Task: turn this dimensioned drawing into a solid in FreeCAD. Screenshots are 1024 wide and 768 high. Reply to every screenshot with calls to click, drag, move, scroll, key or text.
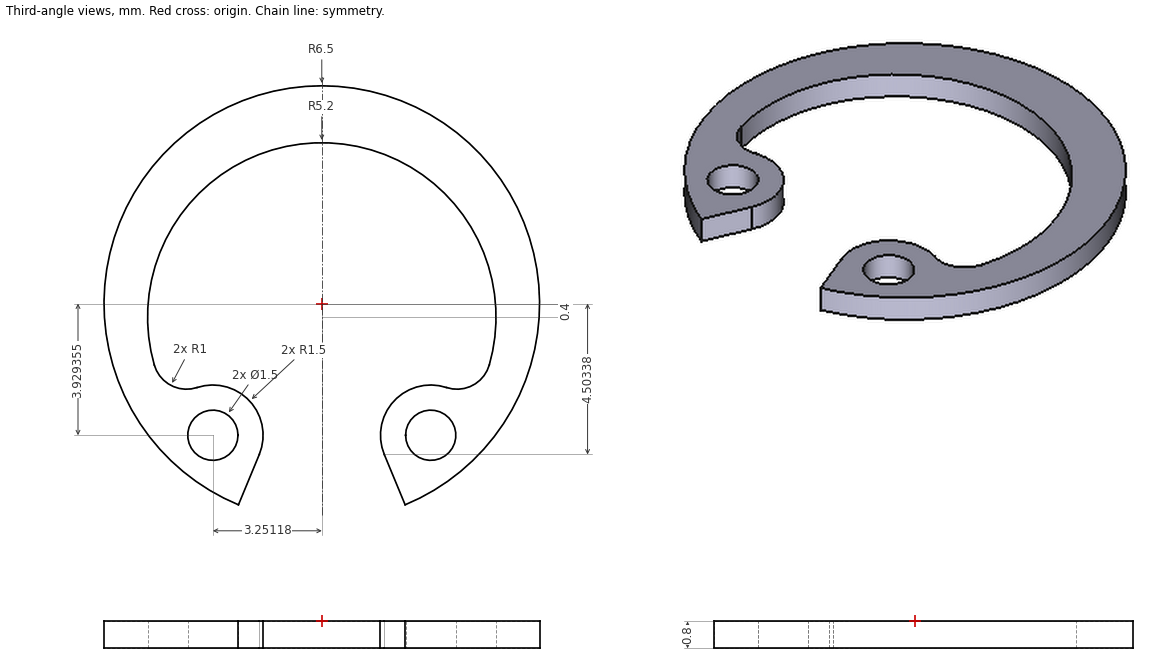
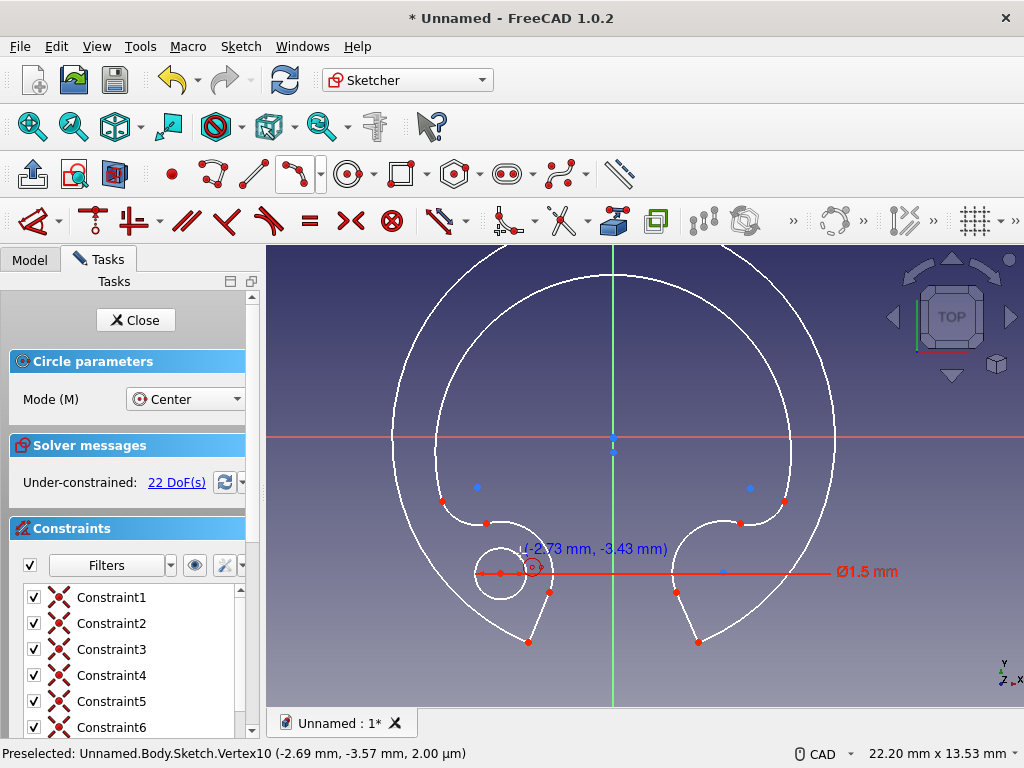
click(724, 571)
move(742, 553)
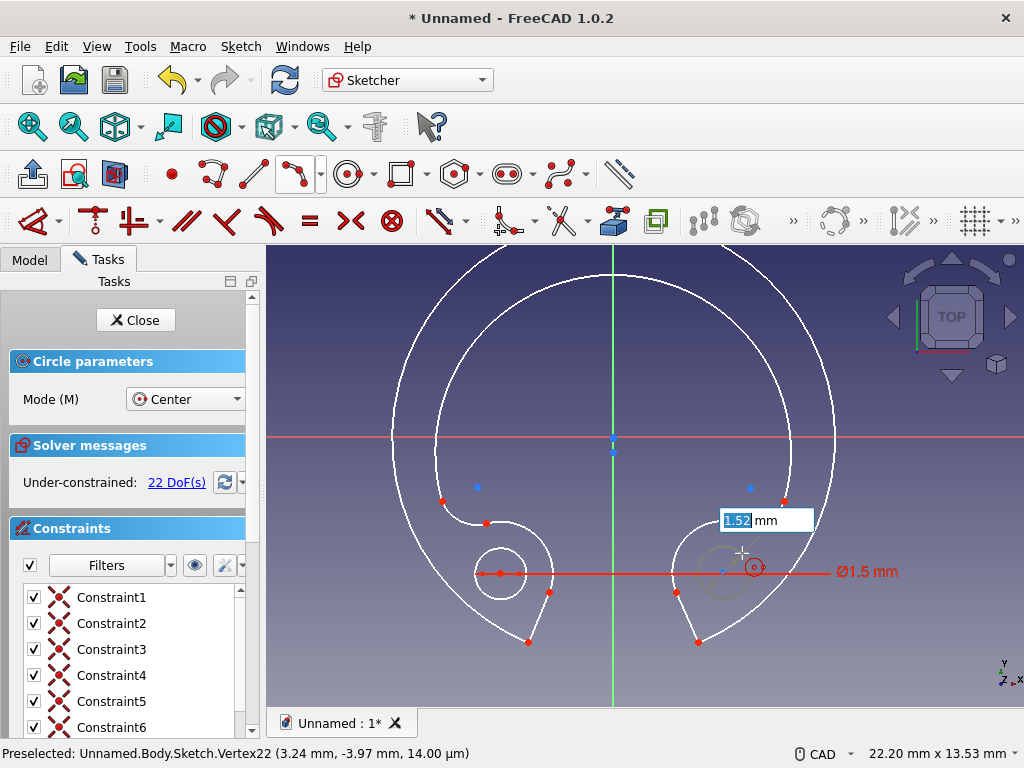
text(1.5)
key(Return)
key(Escape)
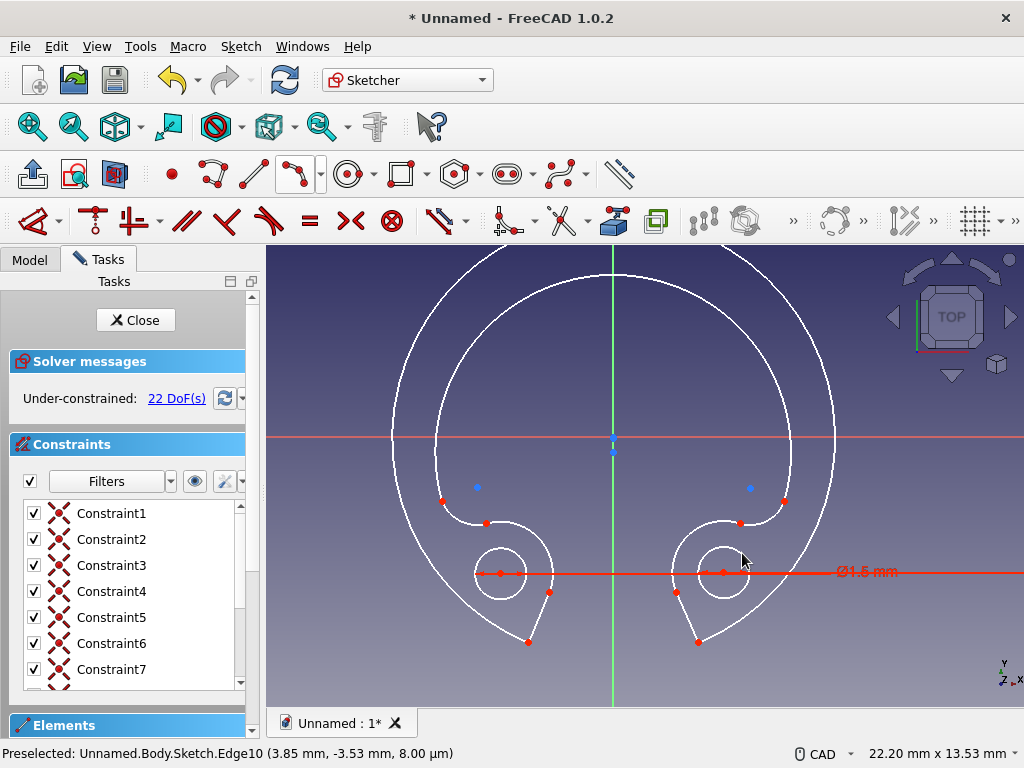
click(683, 607)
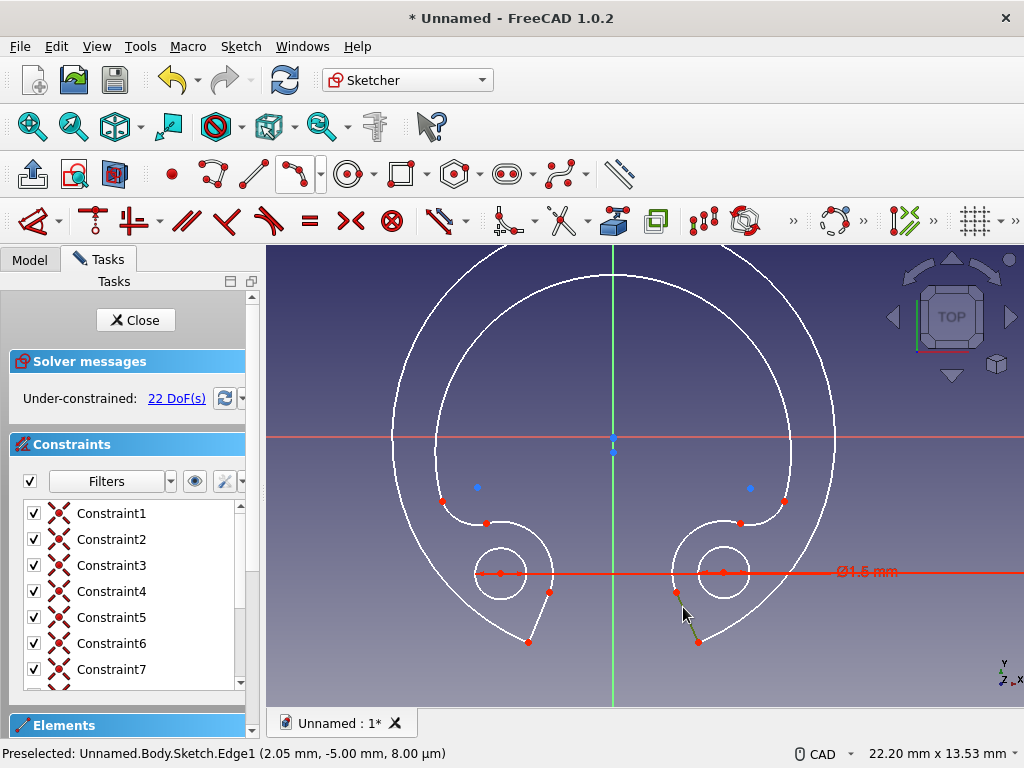
click(706, 524)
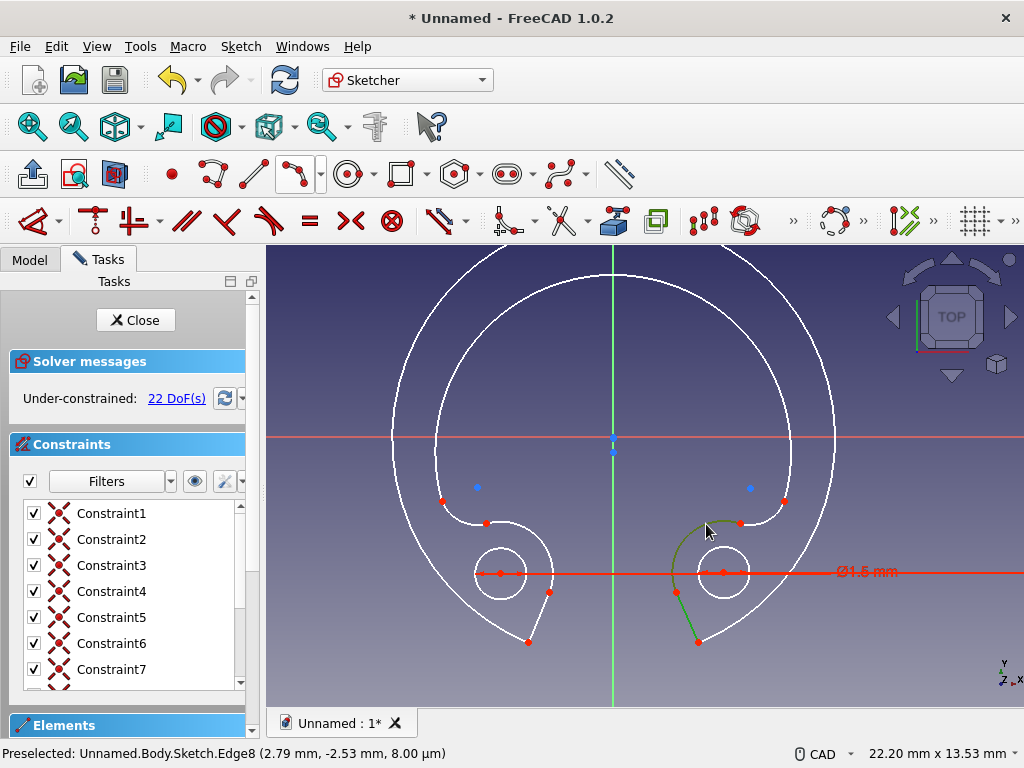
key(t)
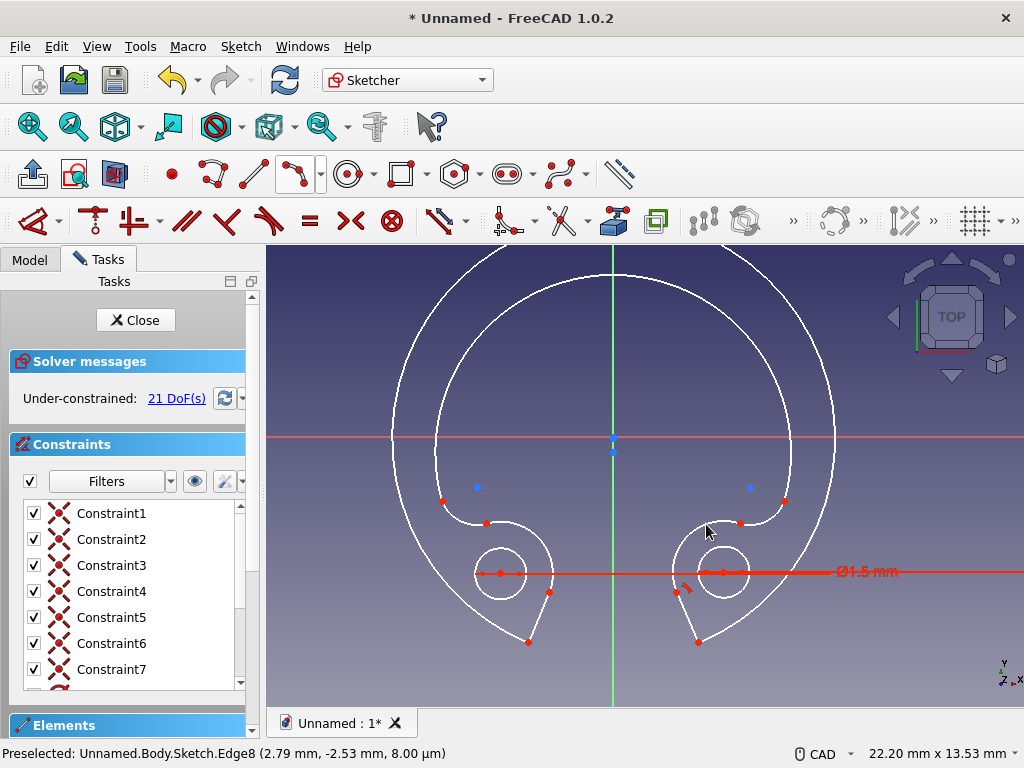
click(535, 628)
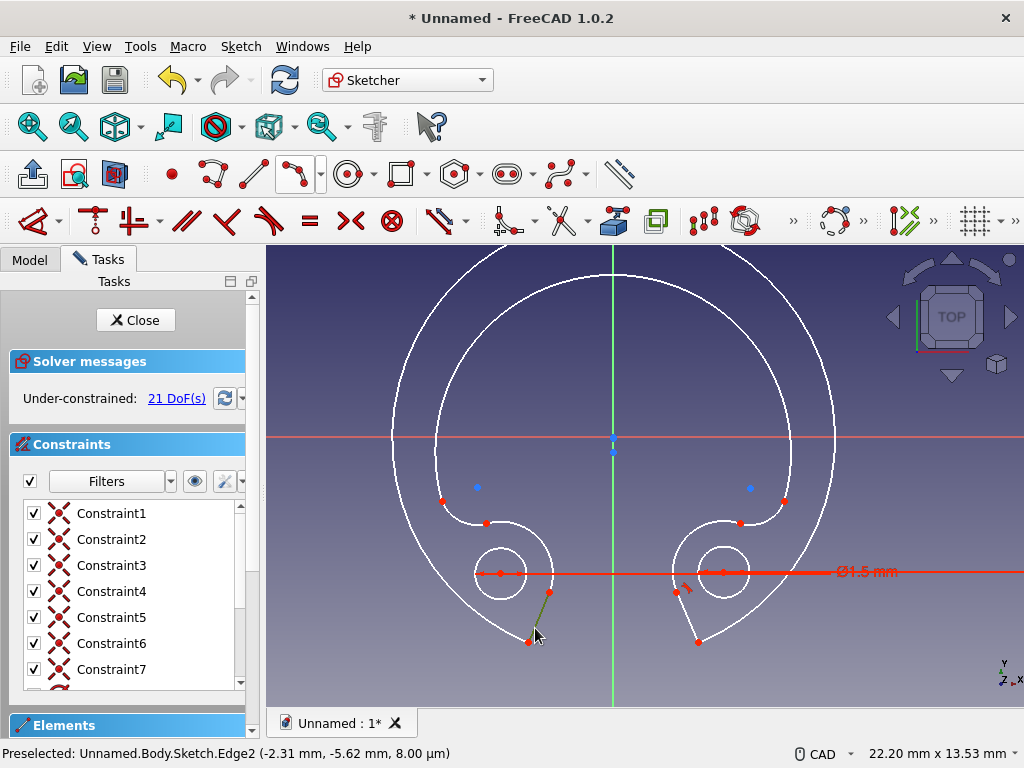
click(551, 558)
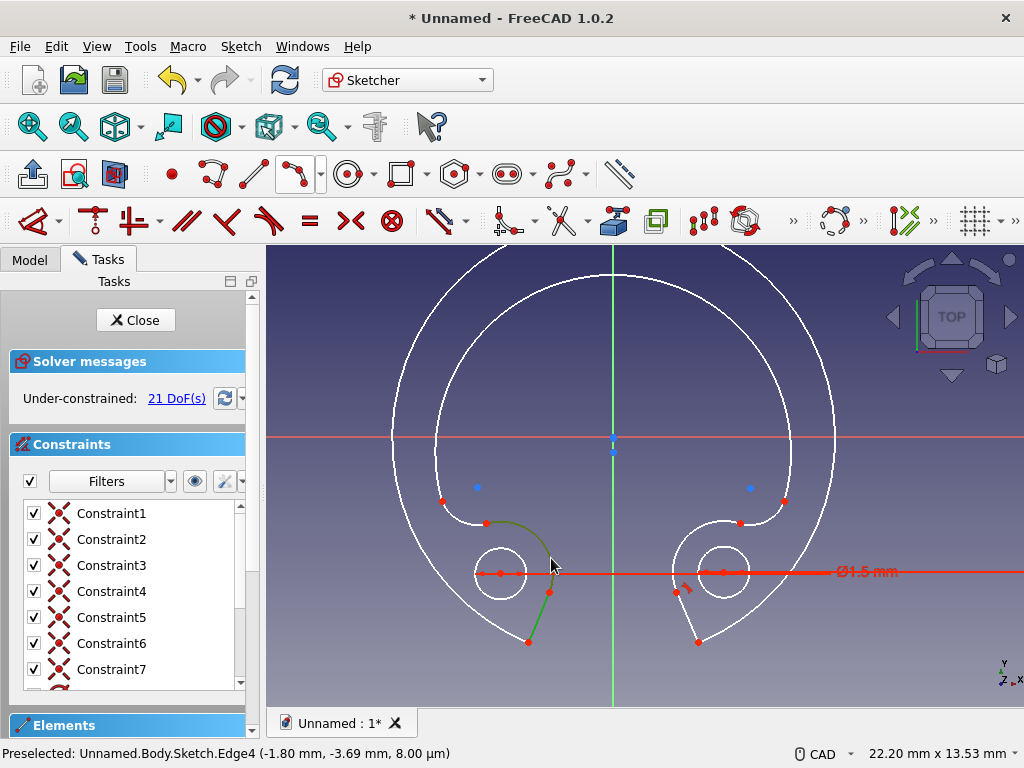
key(t)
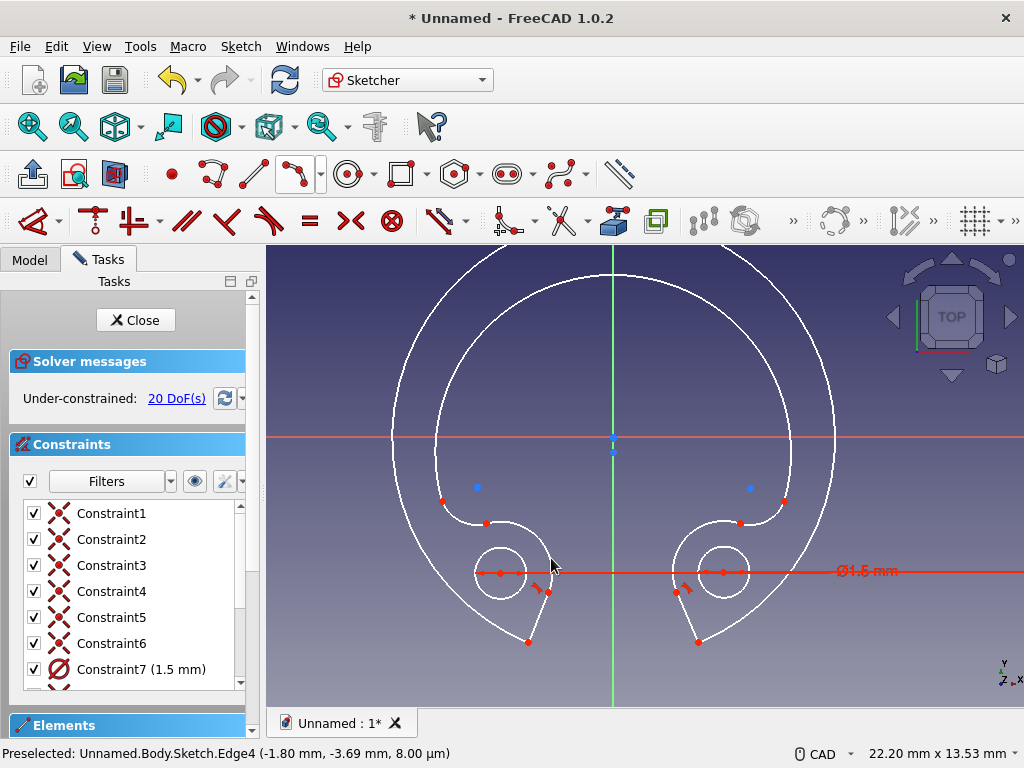
click(550, 559)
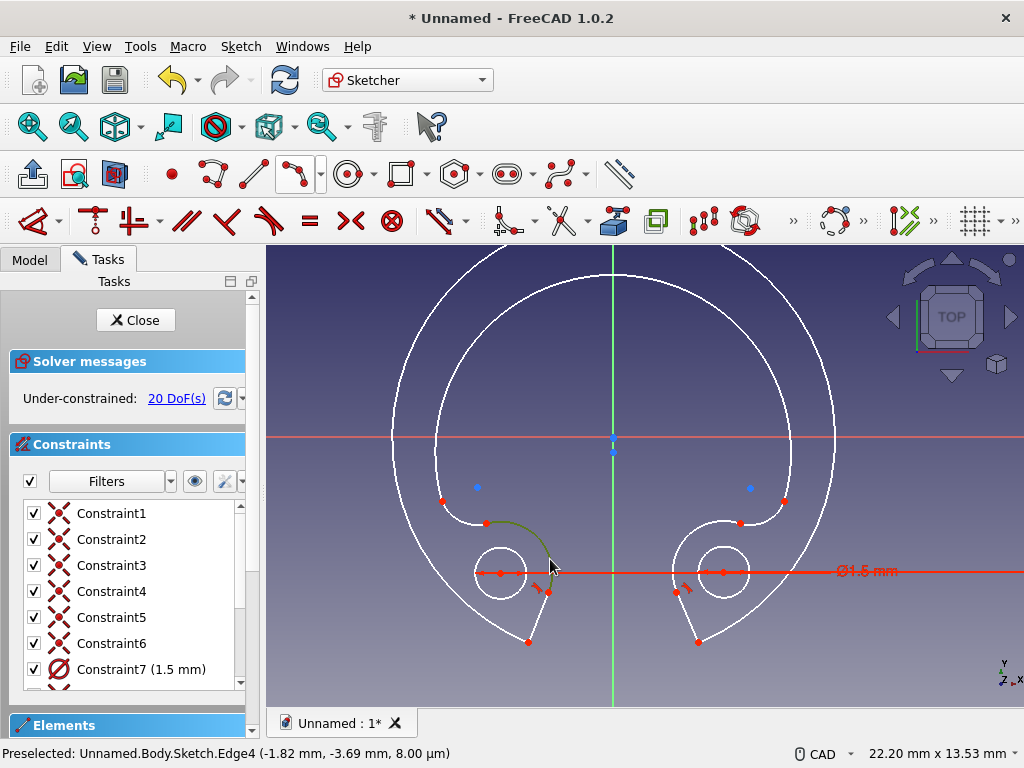
click(451, 515)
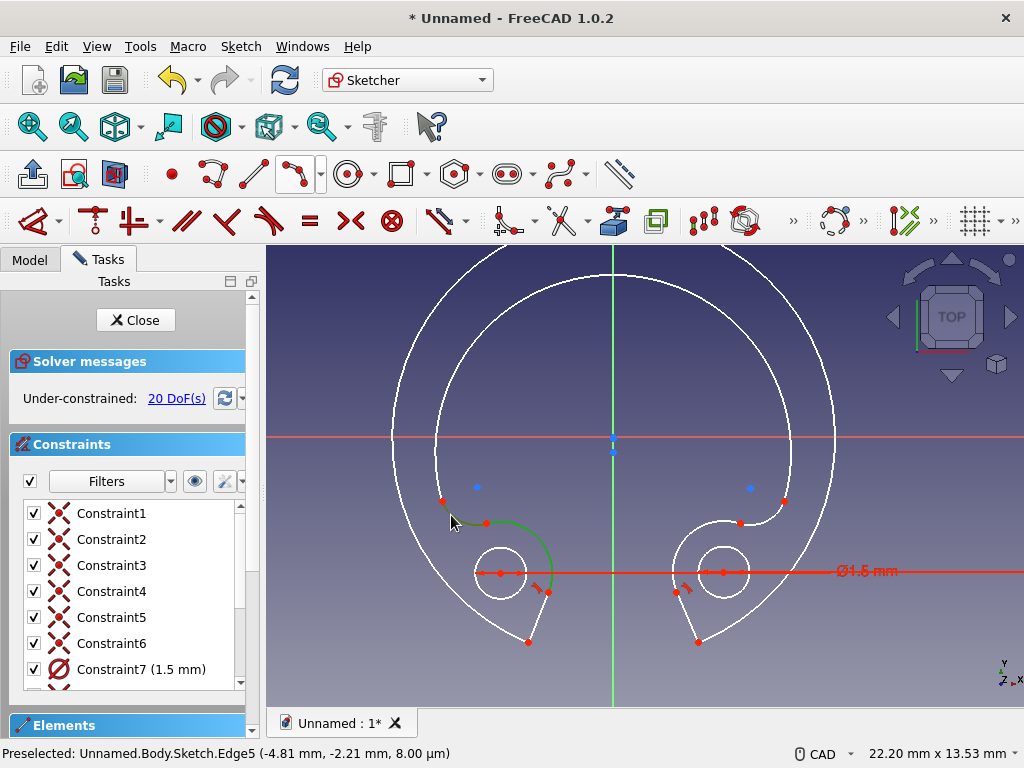
click(269, 222)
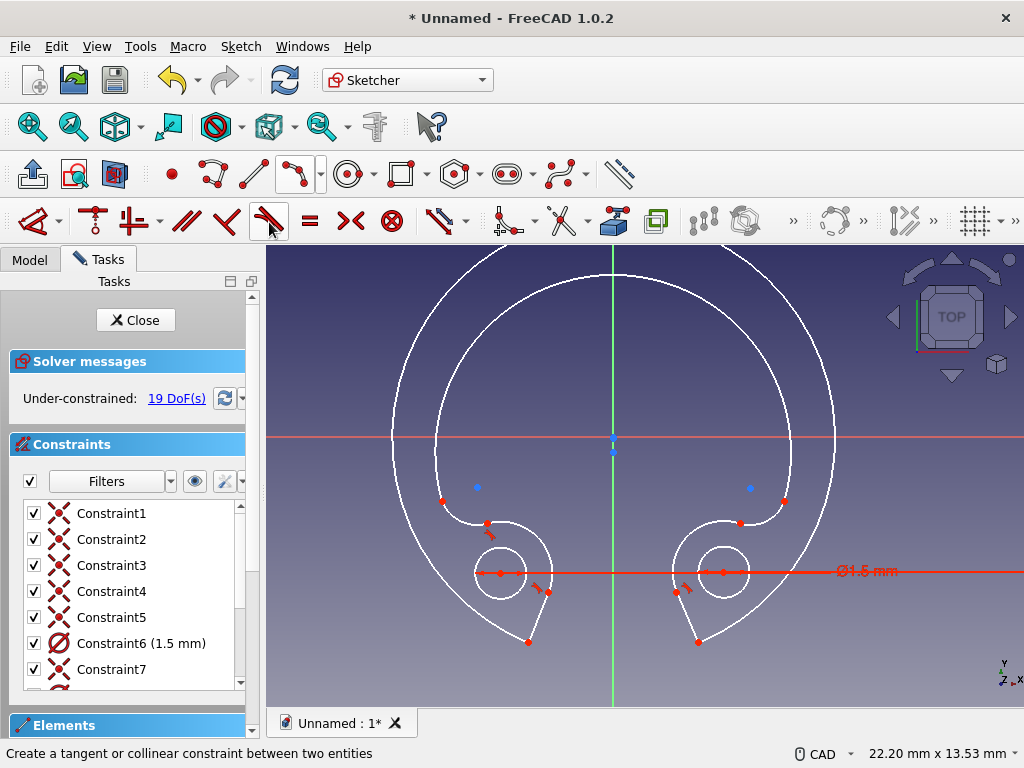
click(451, 515)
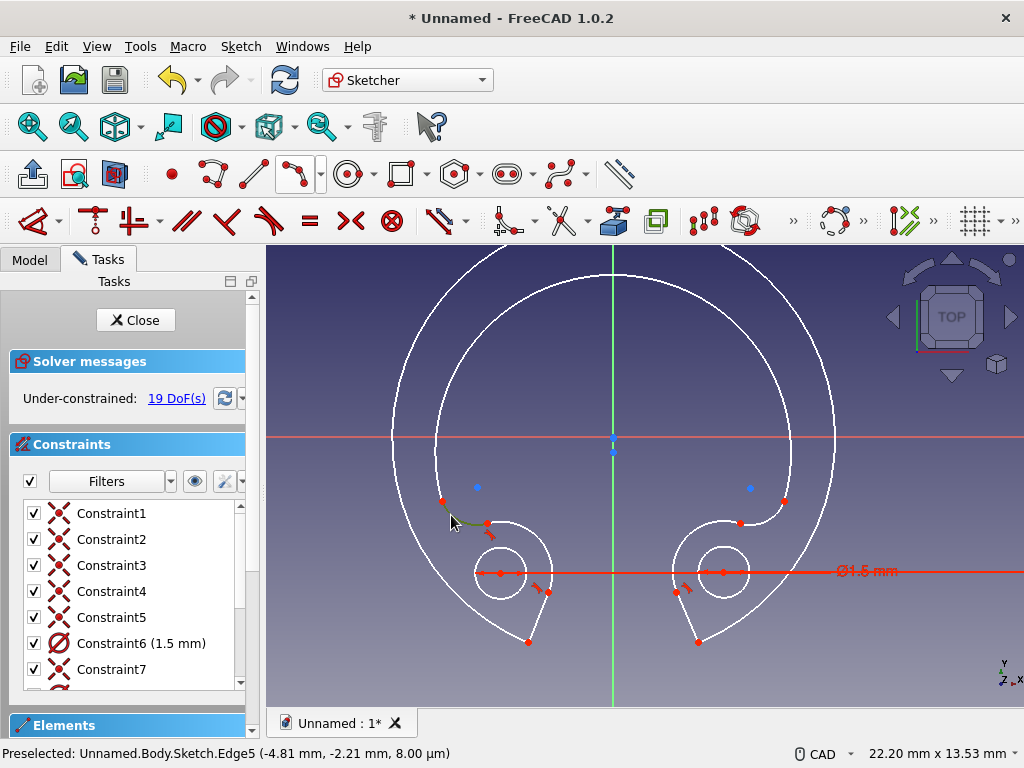
click(733, 321)